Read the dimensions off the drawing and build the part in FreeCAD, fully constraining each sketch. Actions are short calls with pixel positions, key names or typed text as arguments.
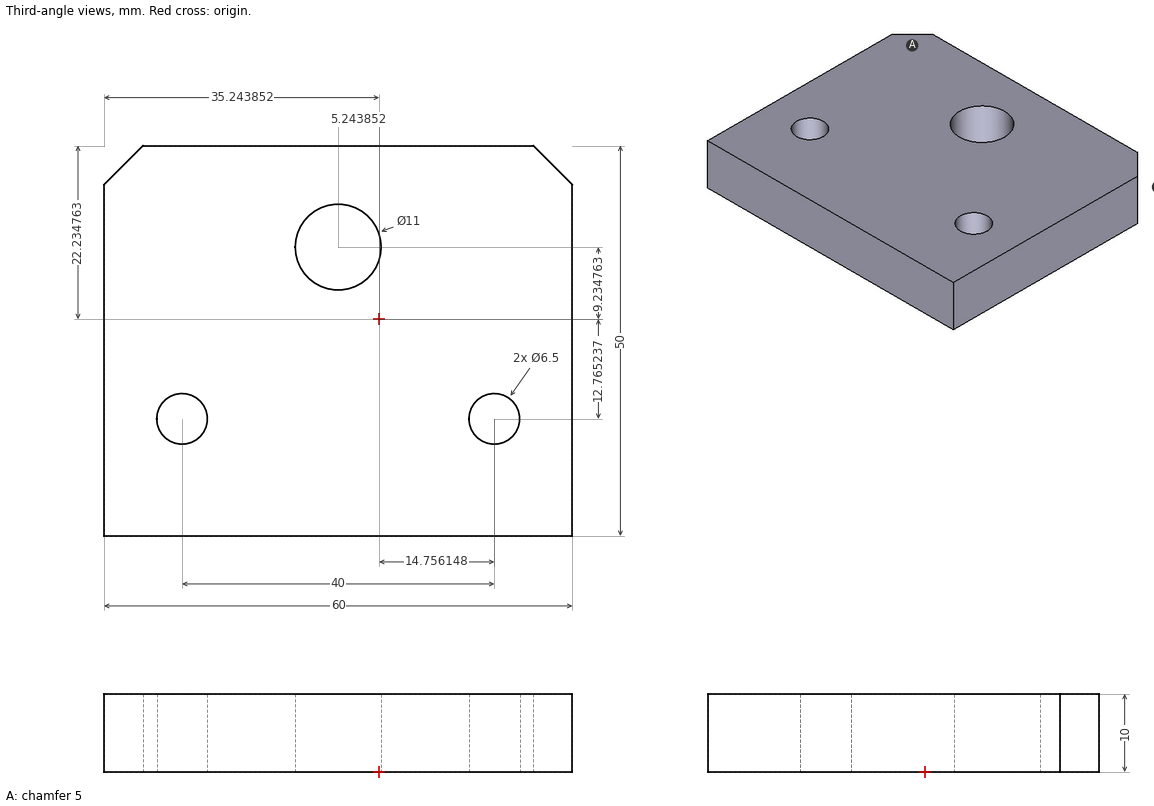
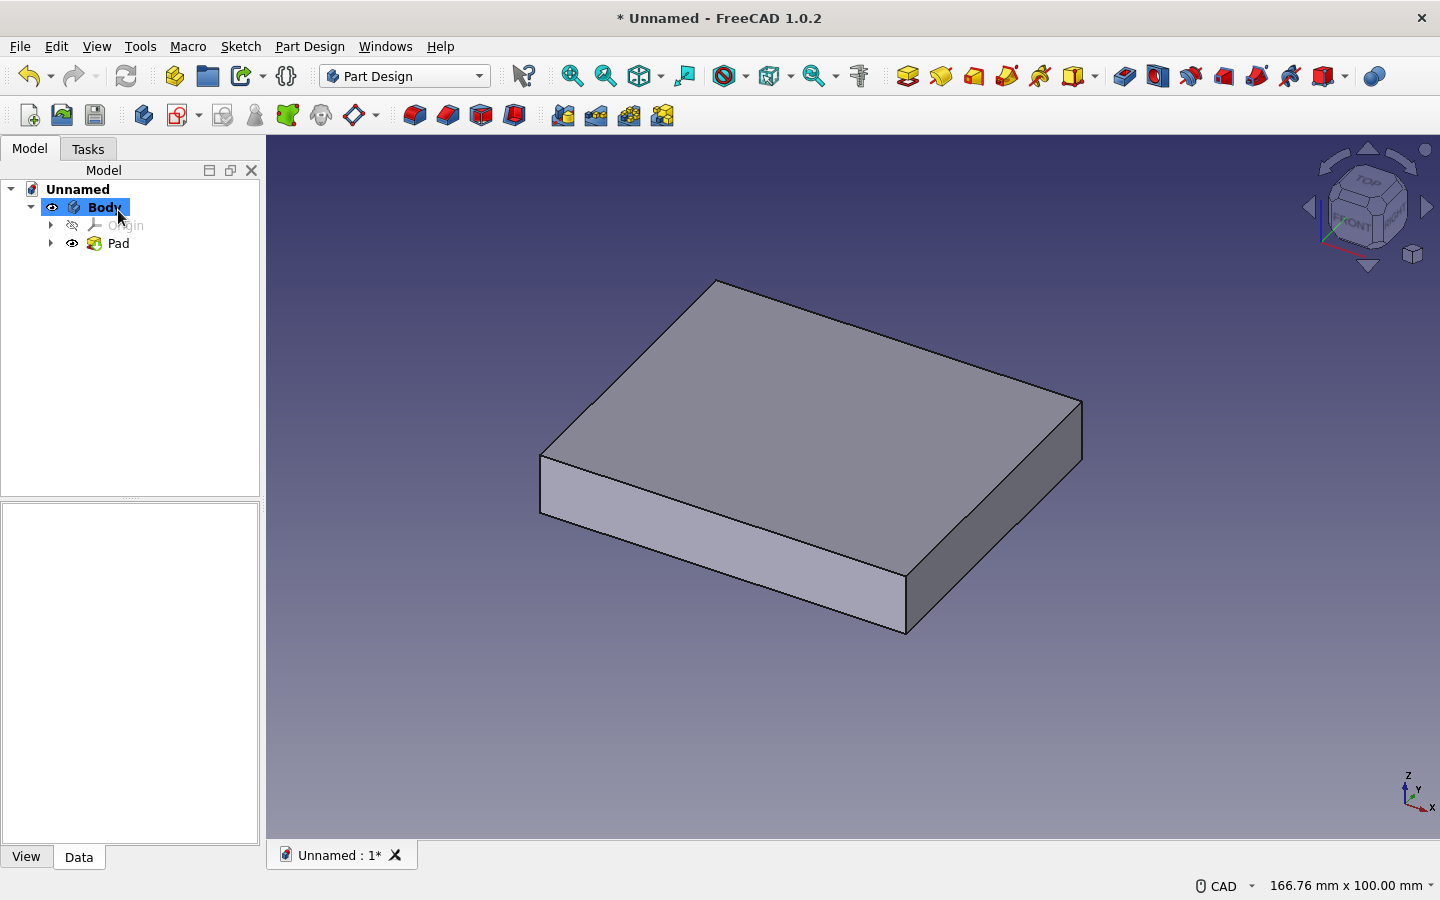
click(176, 116)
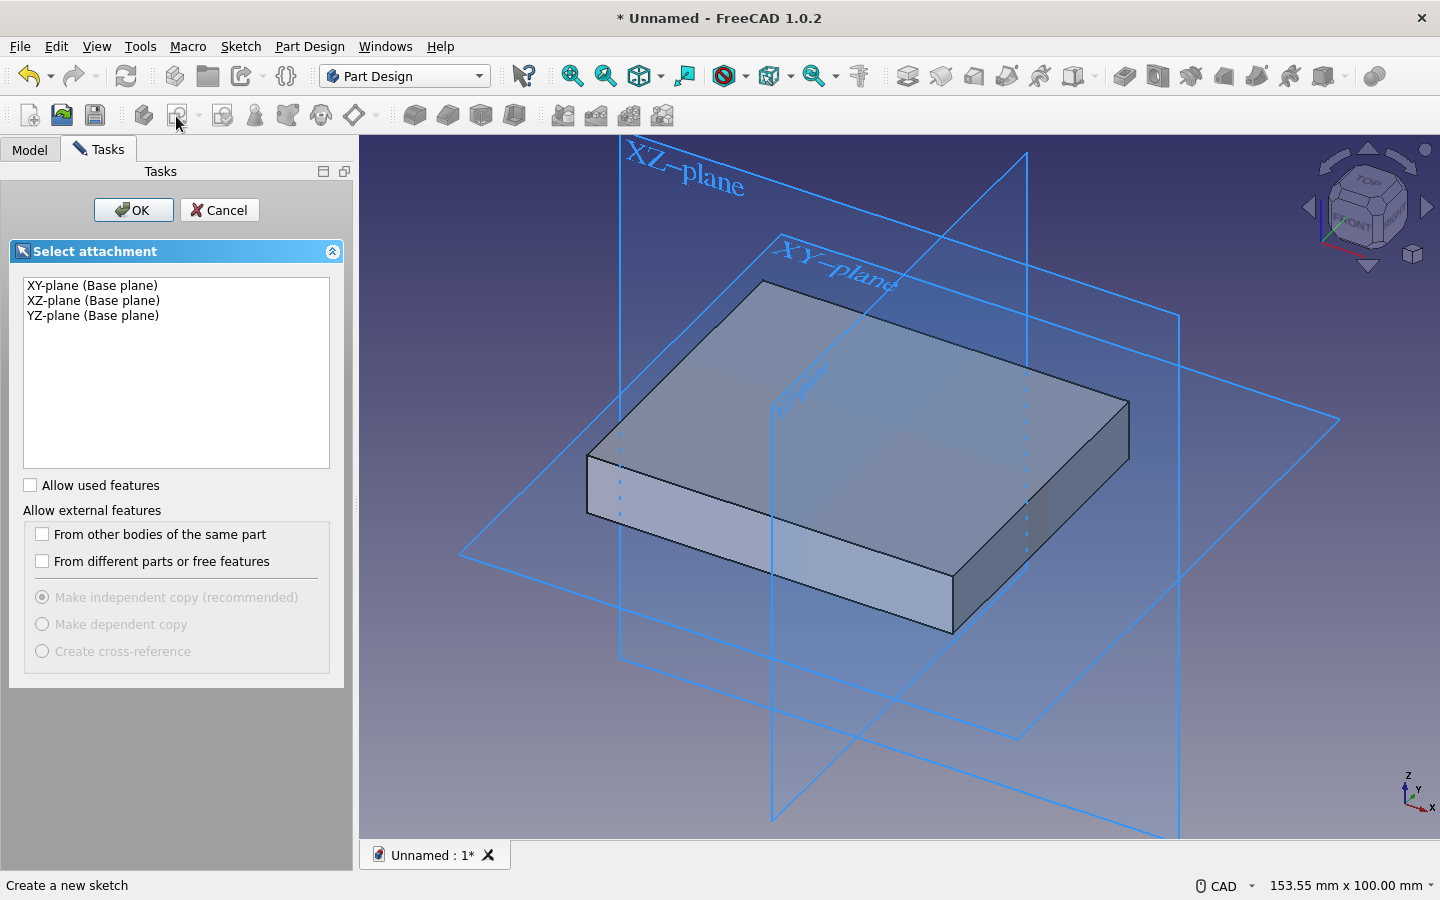
click(84, 286)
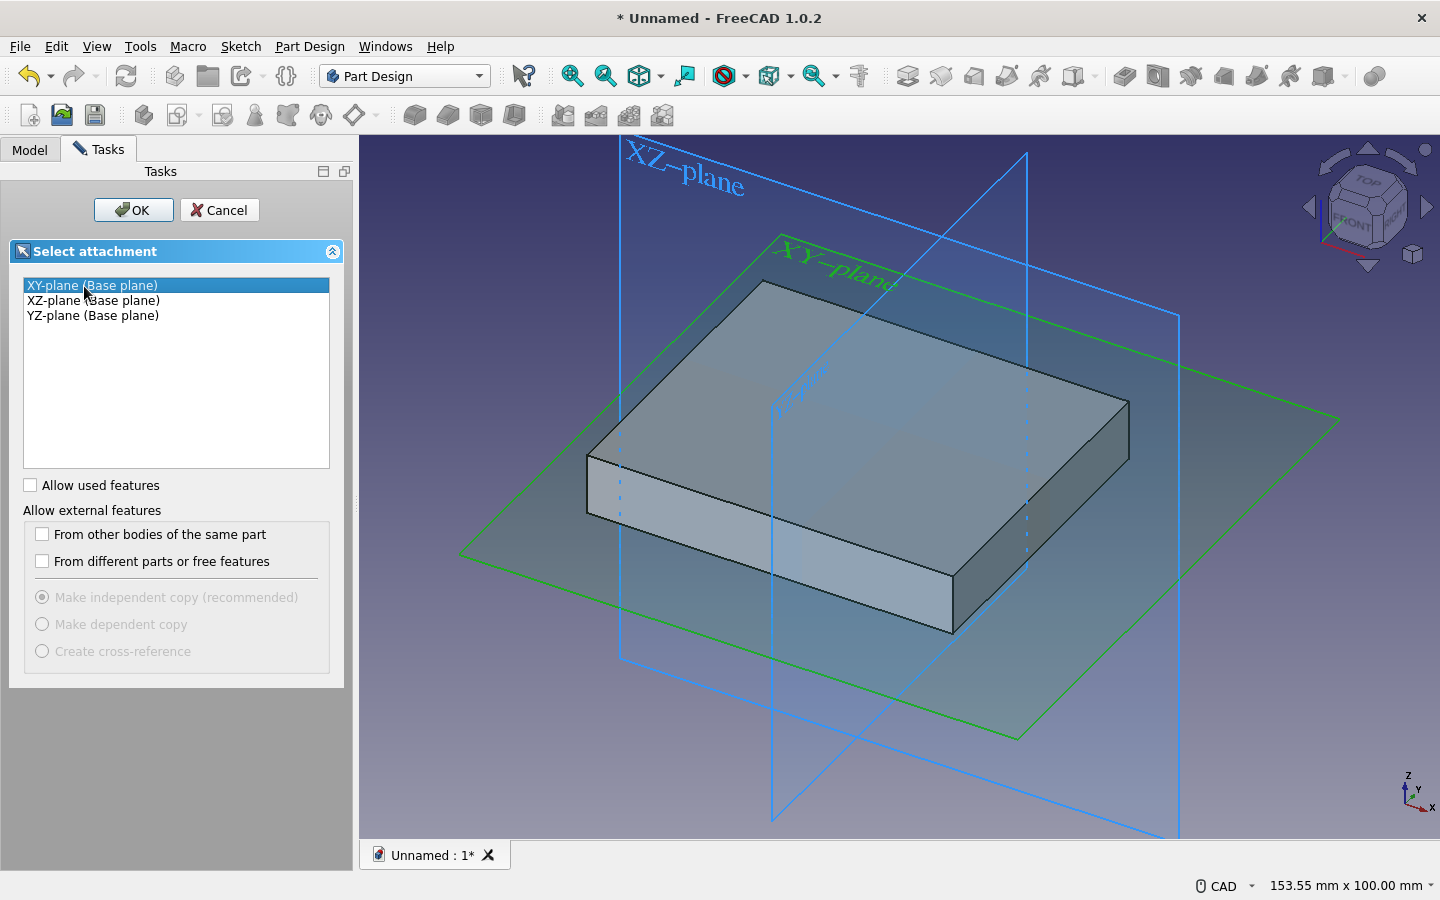
click(134, 210)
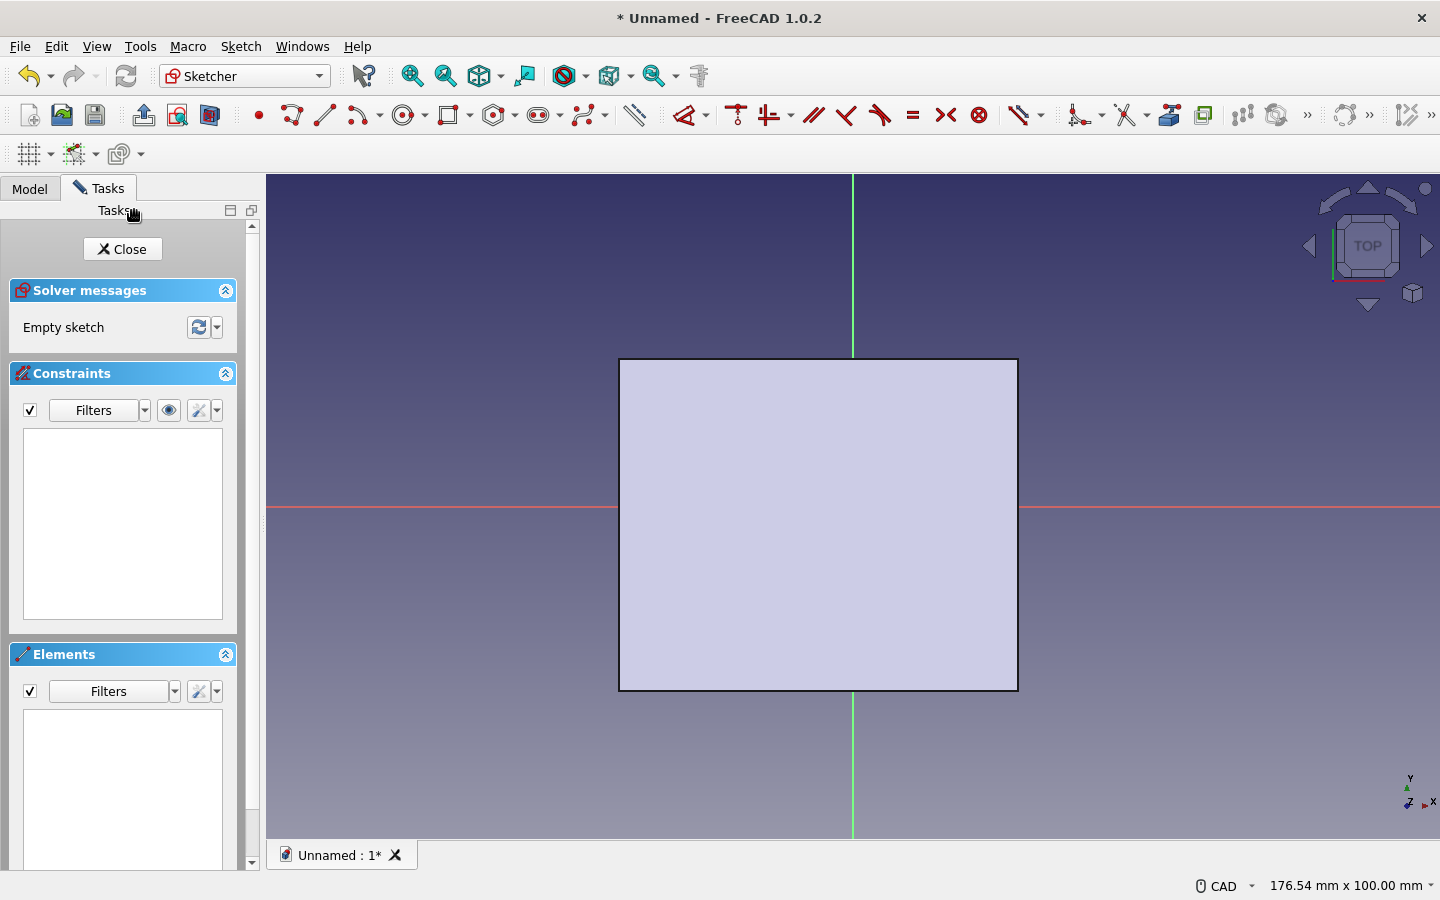
click(210, 116)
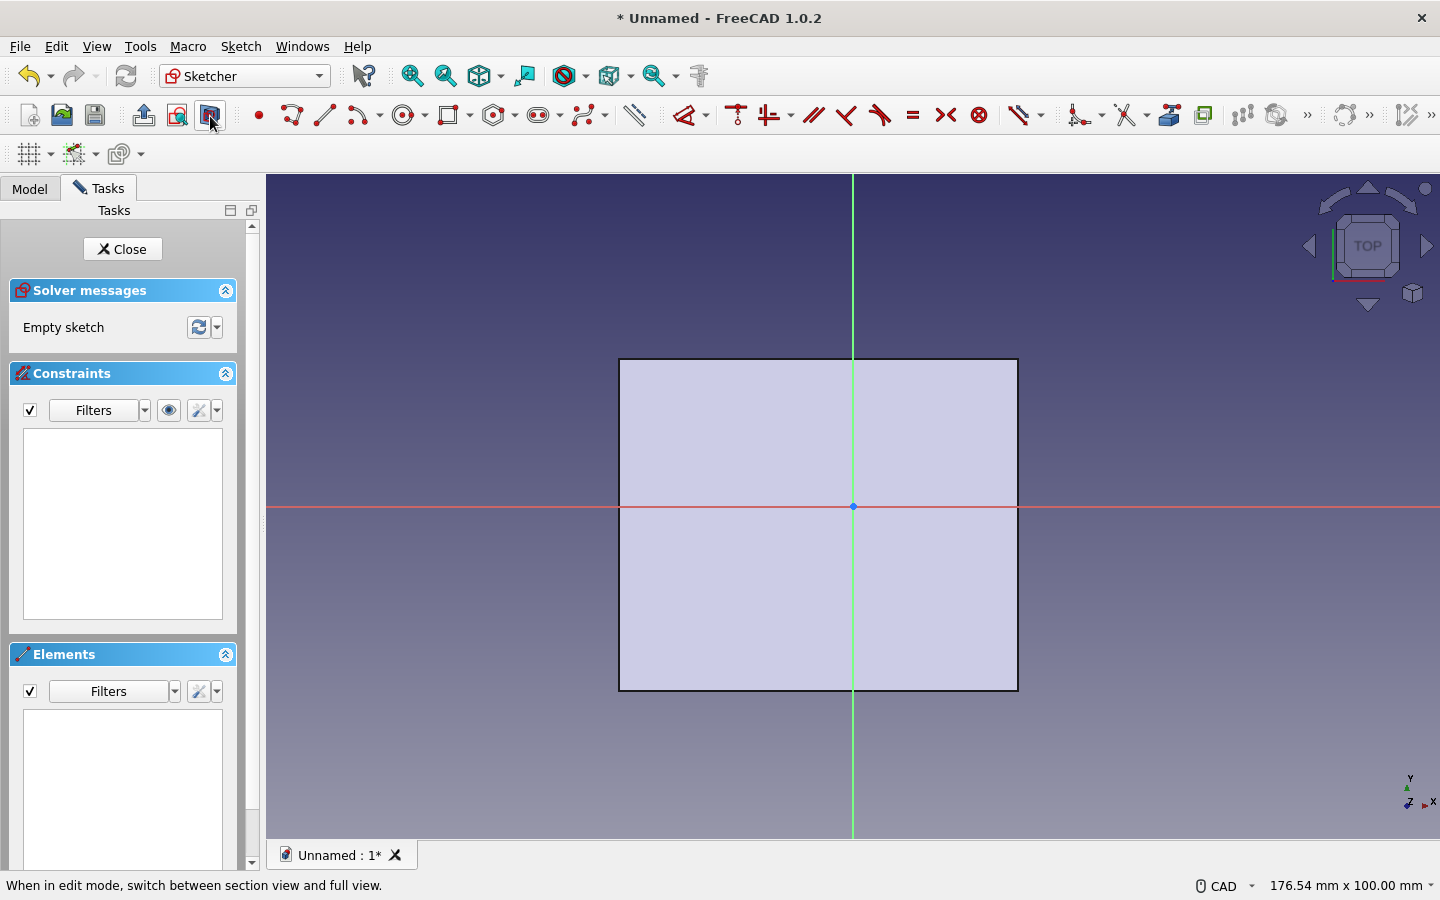
scroll(829, 441, up, 7)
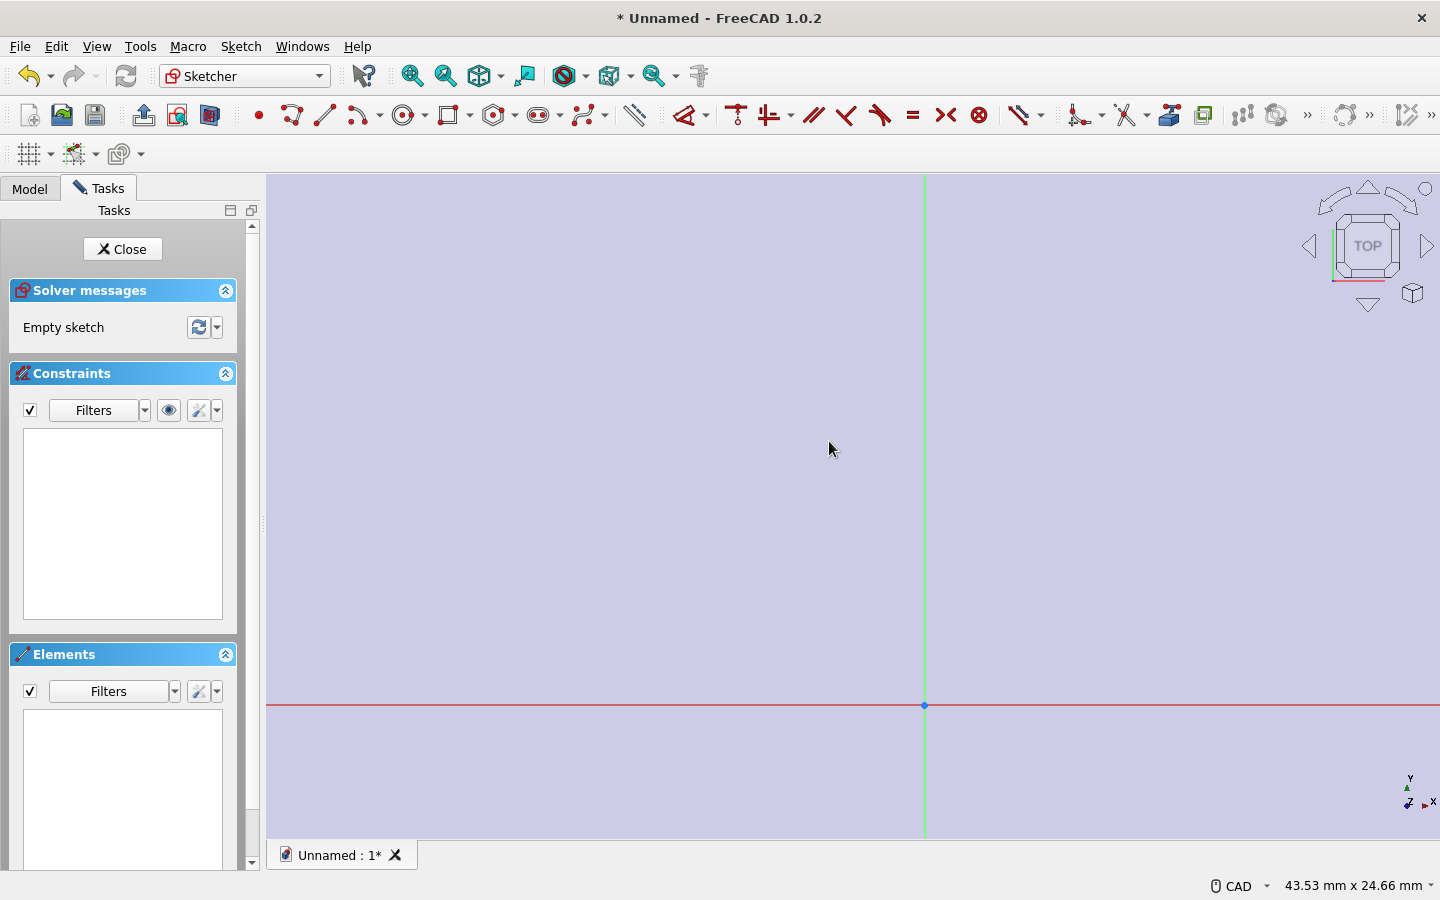
key(g)
key(c)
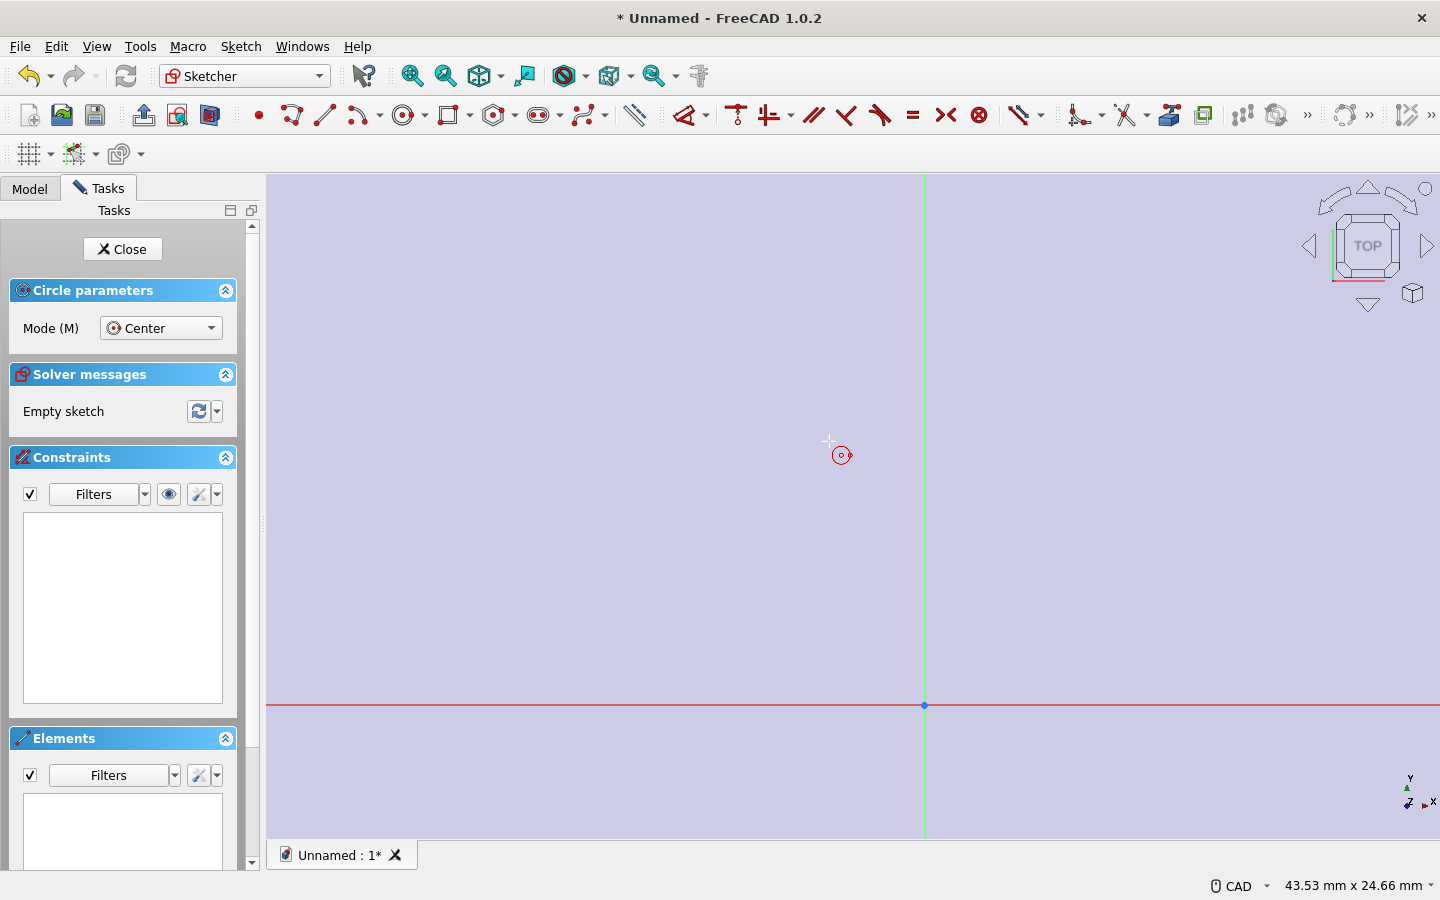
click(783, 456)
move(888, 351)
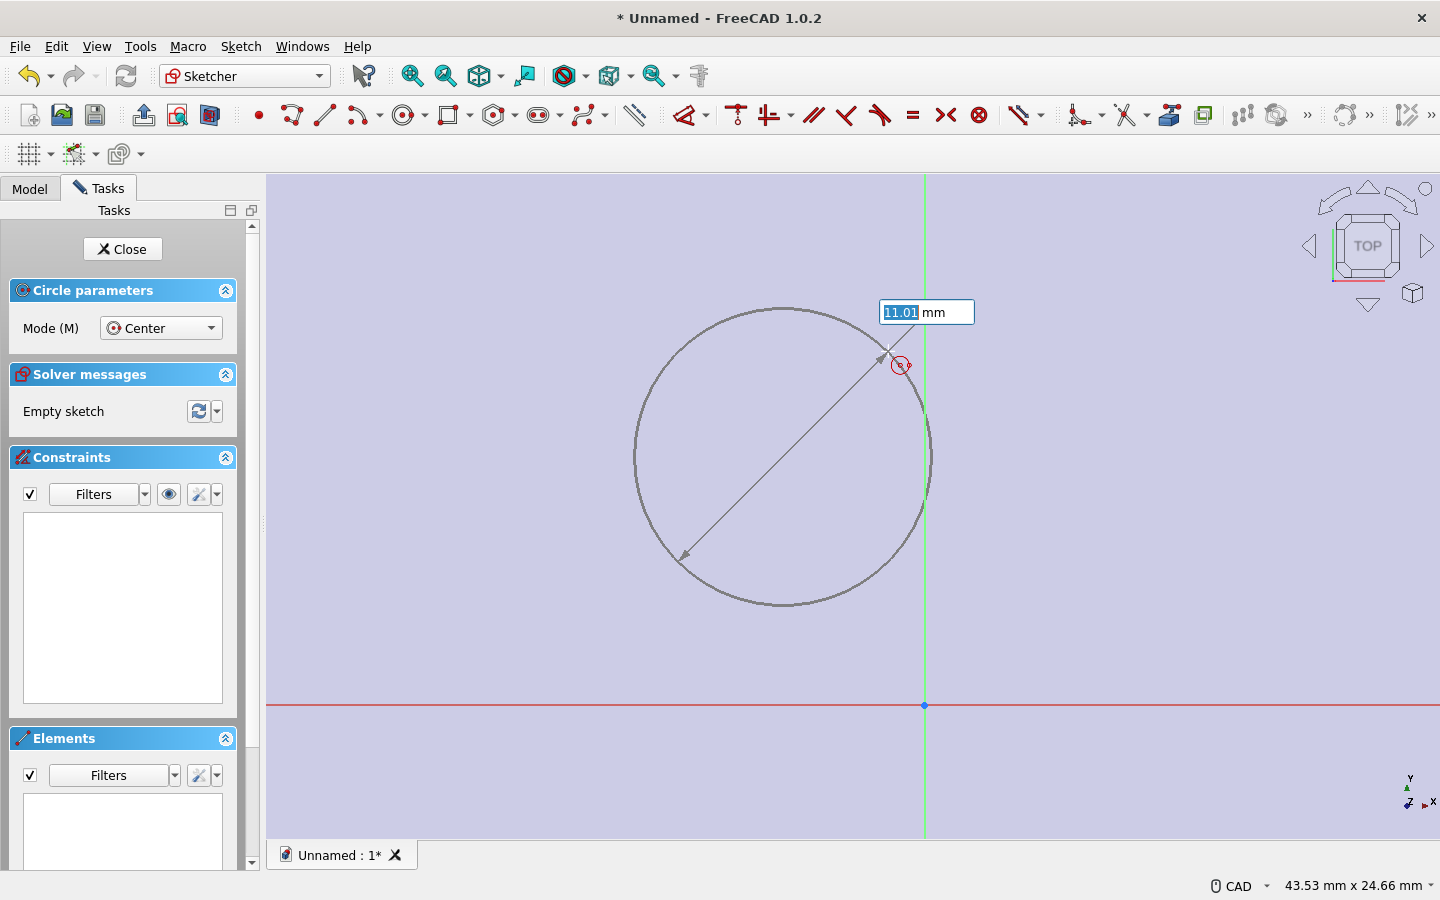
text(11)
key(Return)
key(Escape)